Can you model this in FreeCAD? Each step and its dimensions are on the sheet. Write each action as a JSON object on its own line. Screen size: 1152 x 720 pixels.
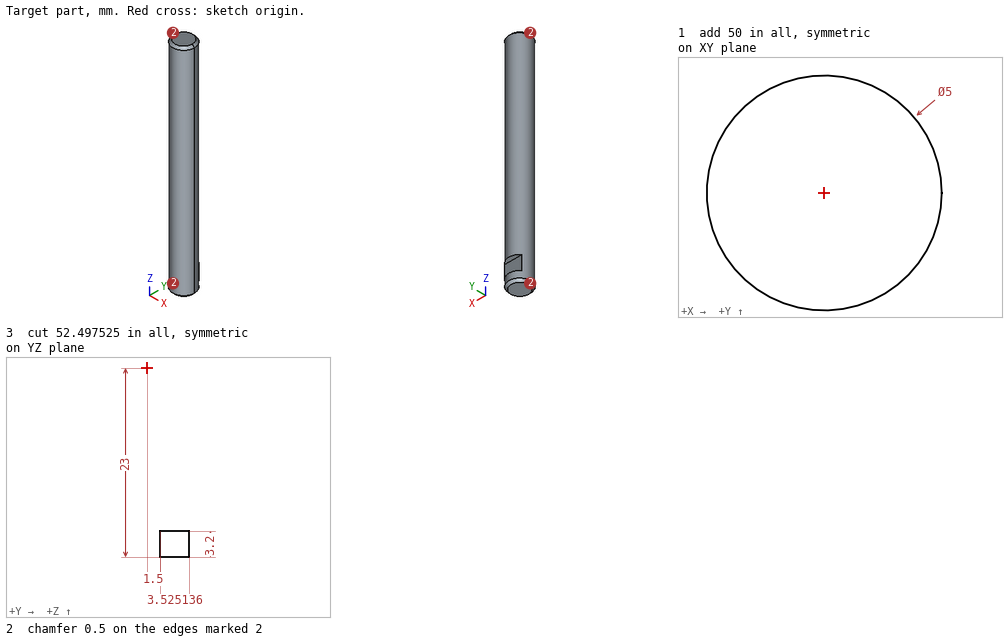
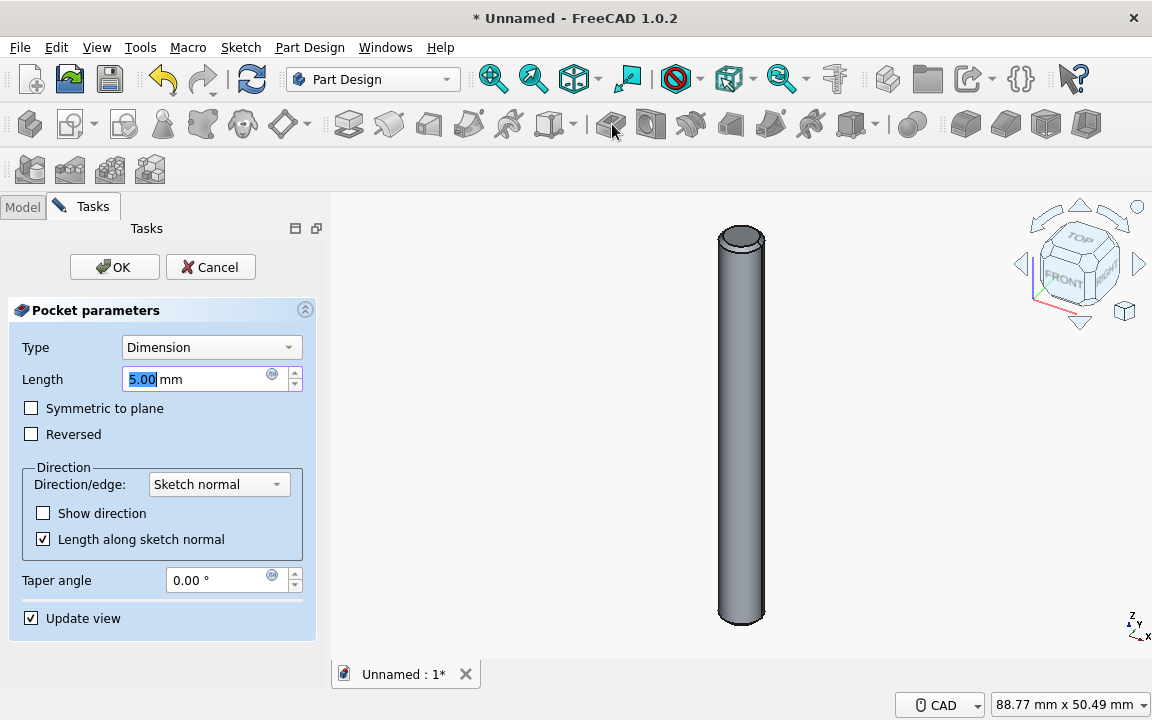
{"action": "type", "text": "52.497525"}
{"action": "key", "text": "Tab"}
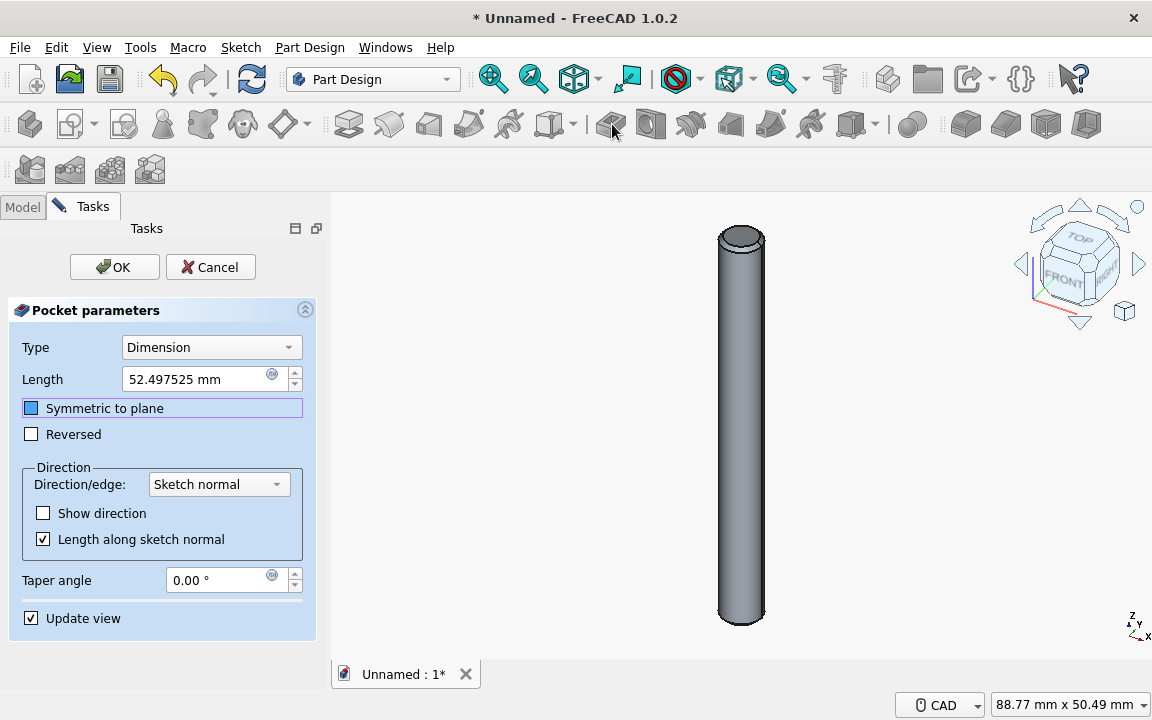
{"action": "left_click", "coordinate": [30, 408]}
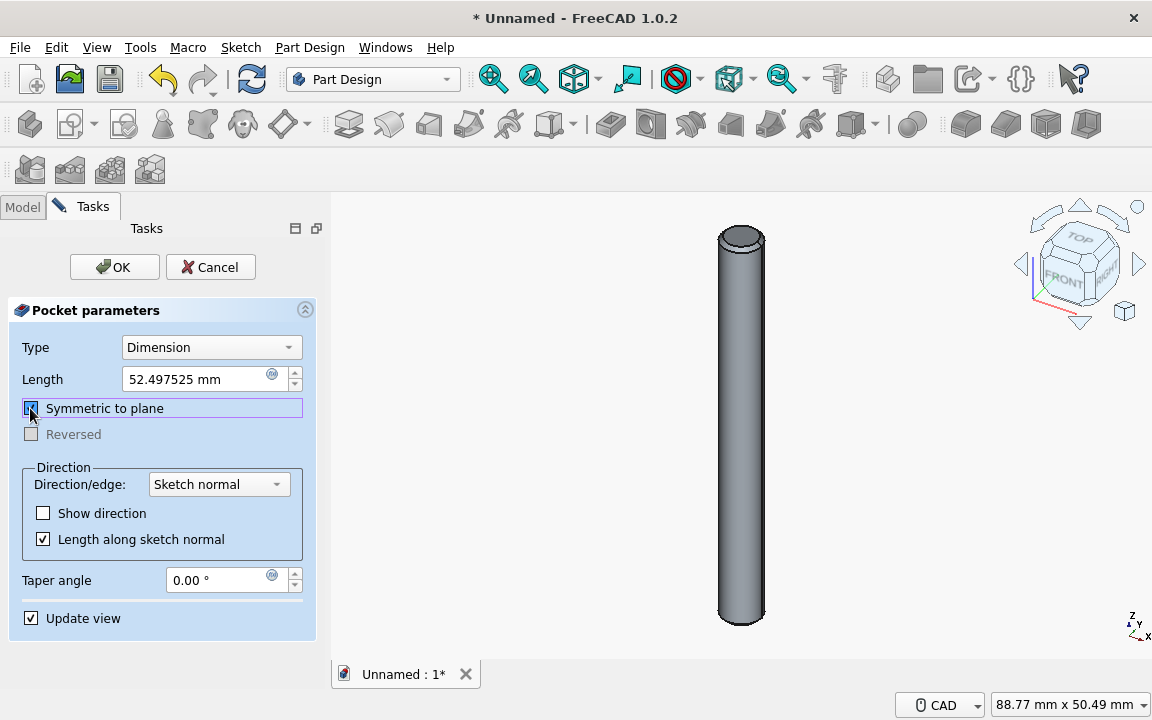
{"action": "left_click", "coordinate": [115, 267]}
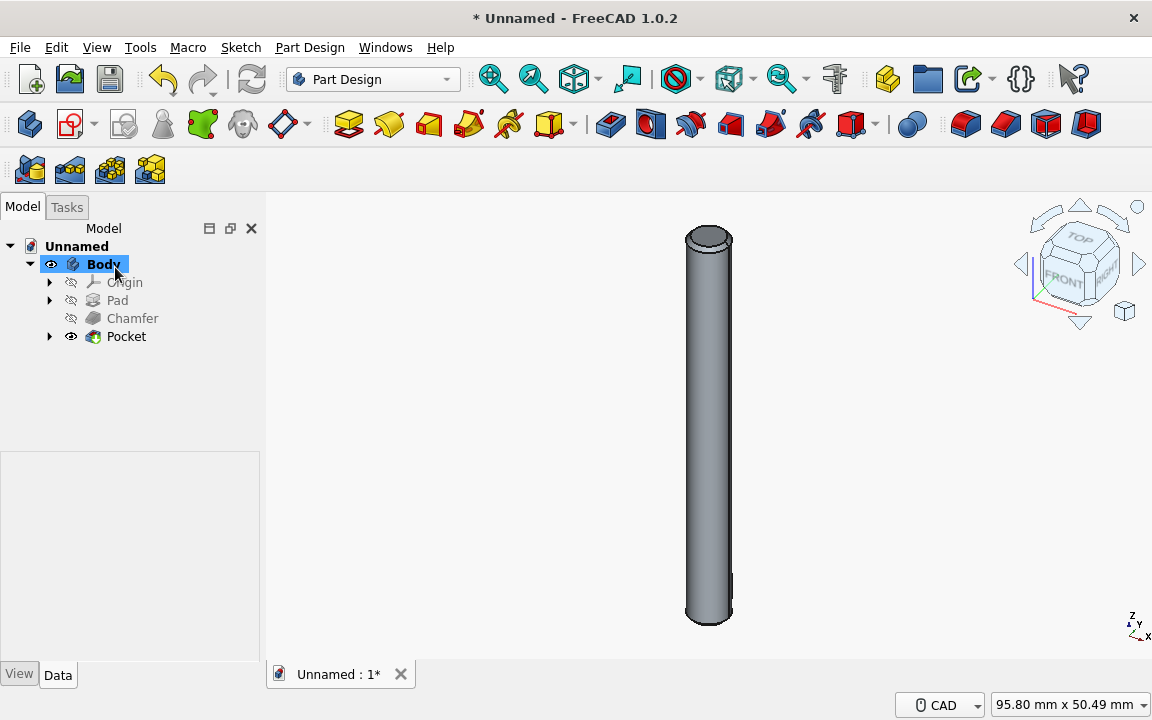
{"action": "key", "text": "0"}